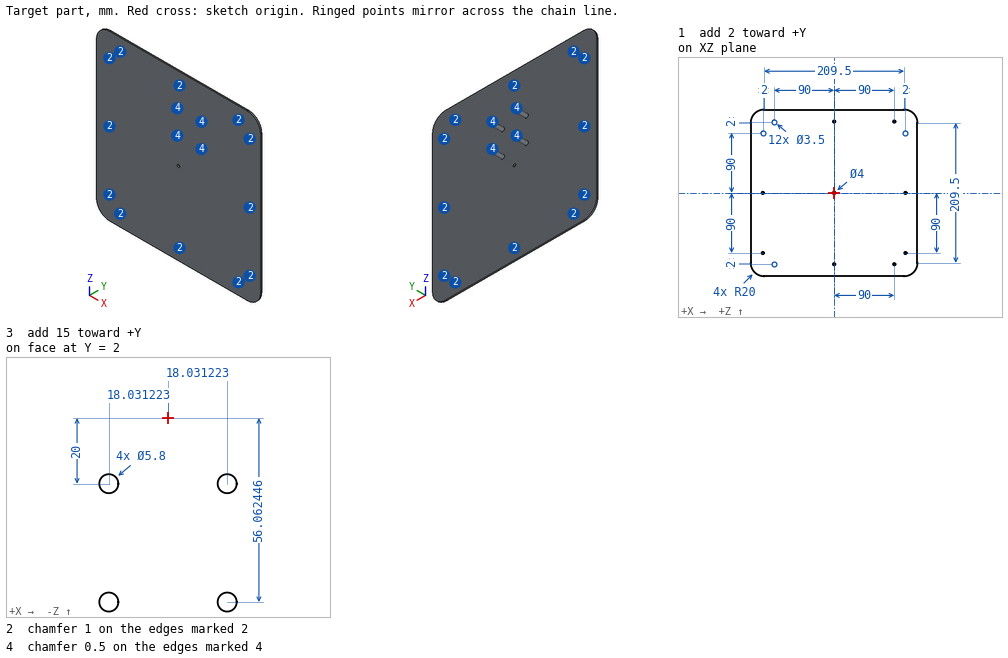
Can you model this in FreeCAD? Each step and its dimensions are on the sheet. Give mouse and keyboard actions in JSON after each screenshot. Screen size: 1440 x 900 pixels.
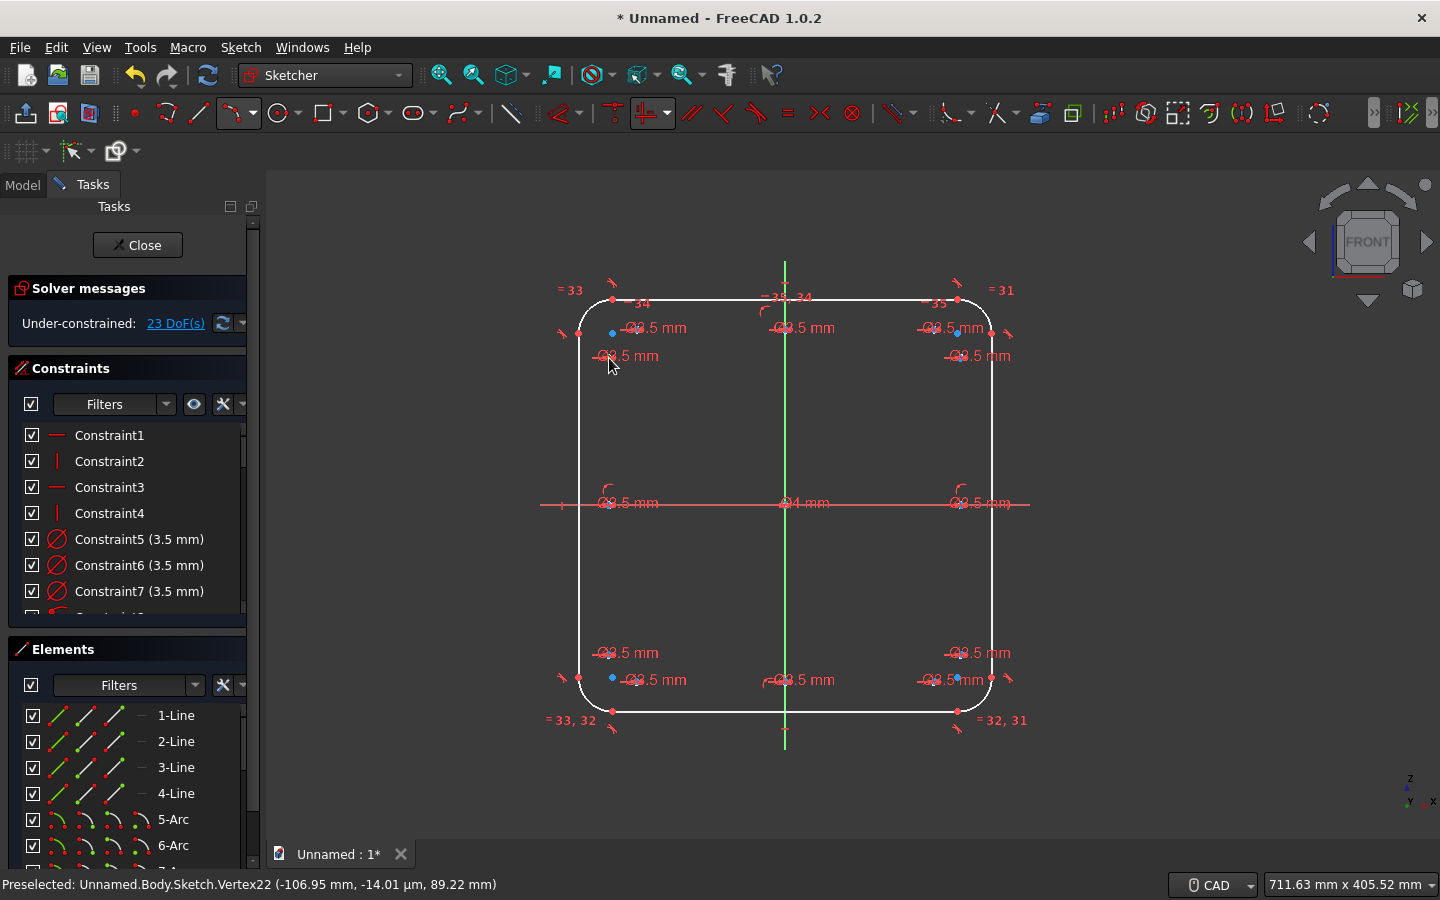
{"action": "left_click", "coordinate": [609, 505]}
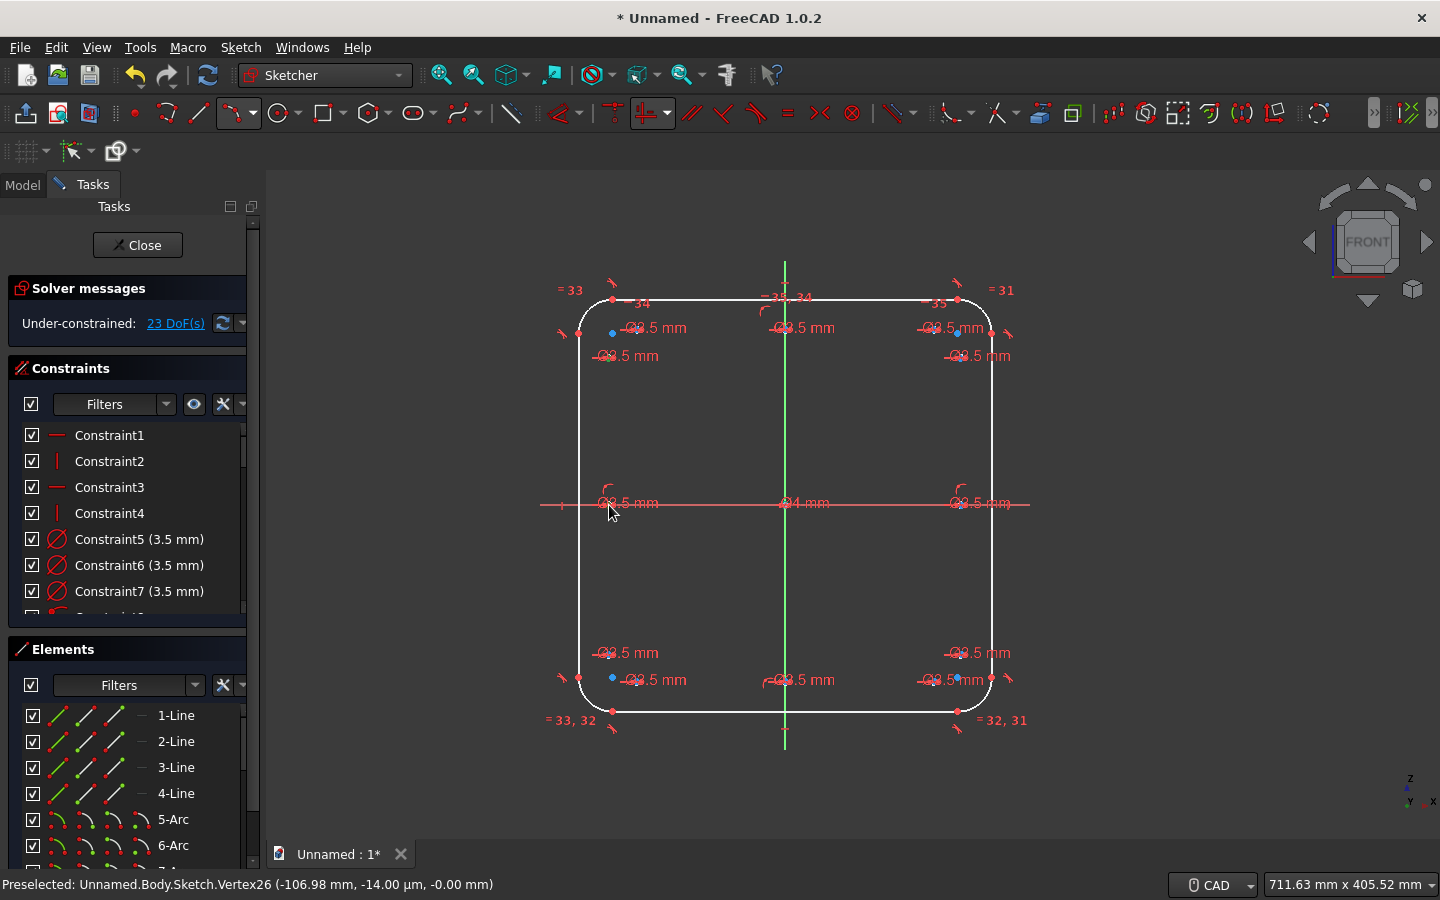
{"action": "left_click", "coordinate": [670, 114]}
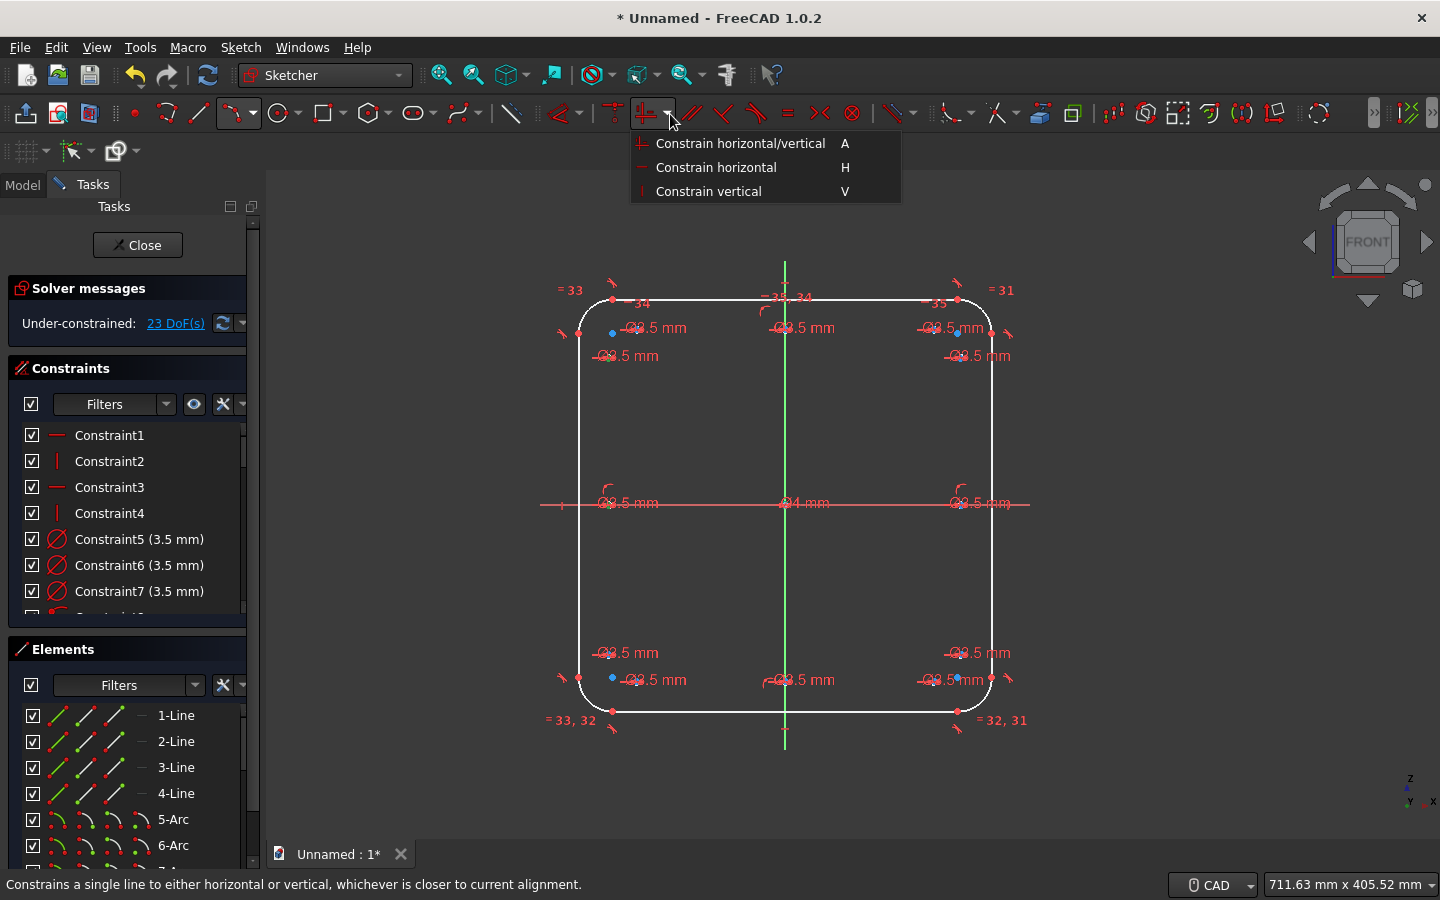
{"action": "left_click", "coordinate": [766, 191]}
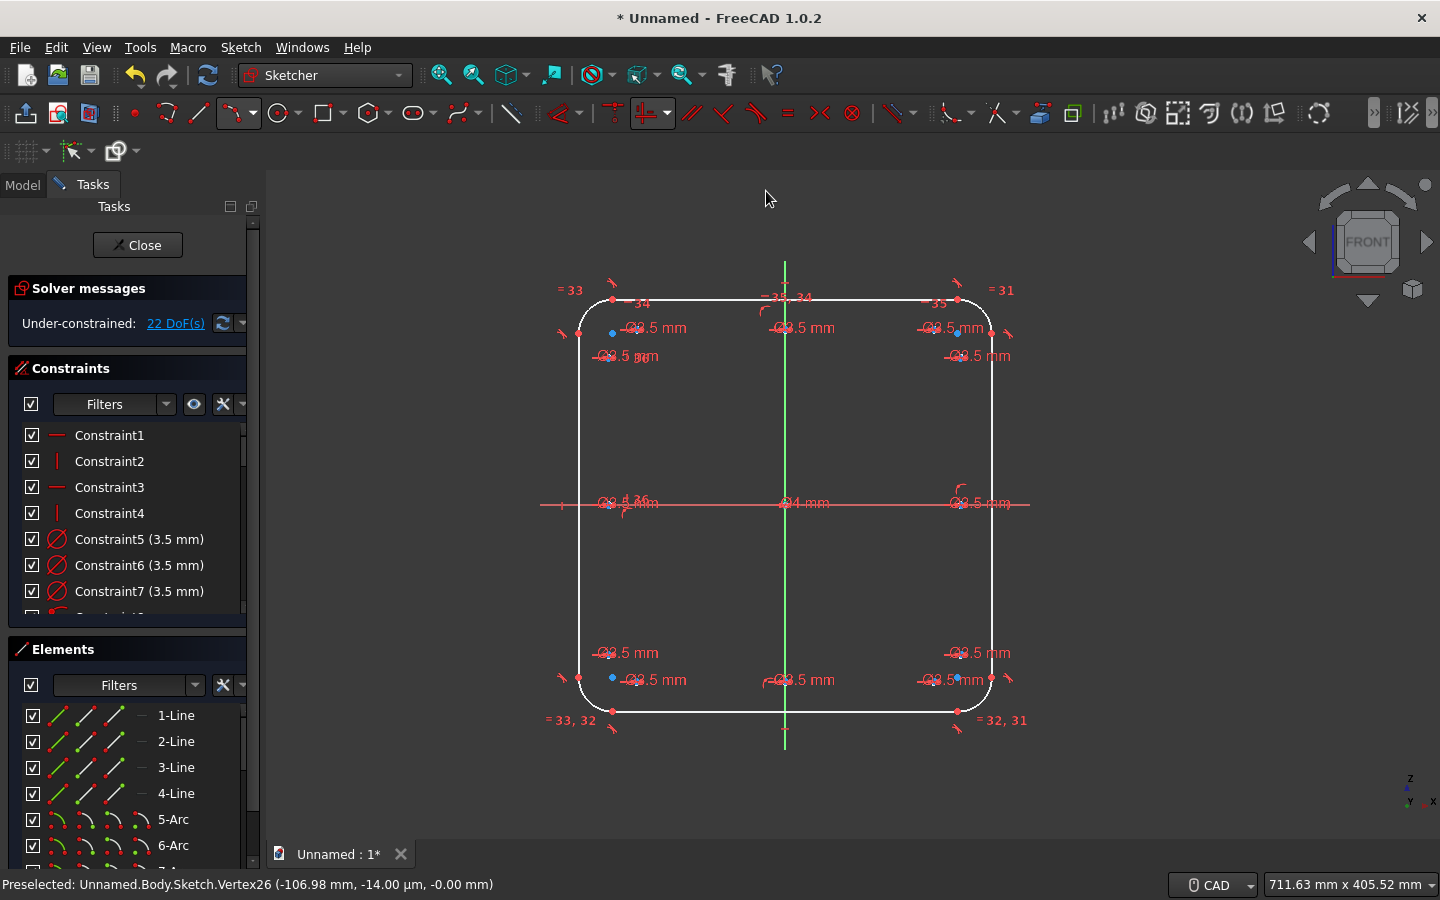
{"action": "left_click", "coordinate": [609, 505]}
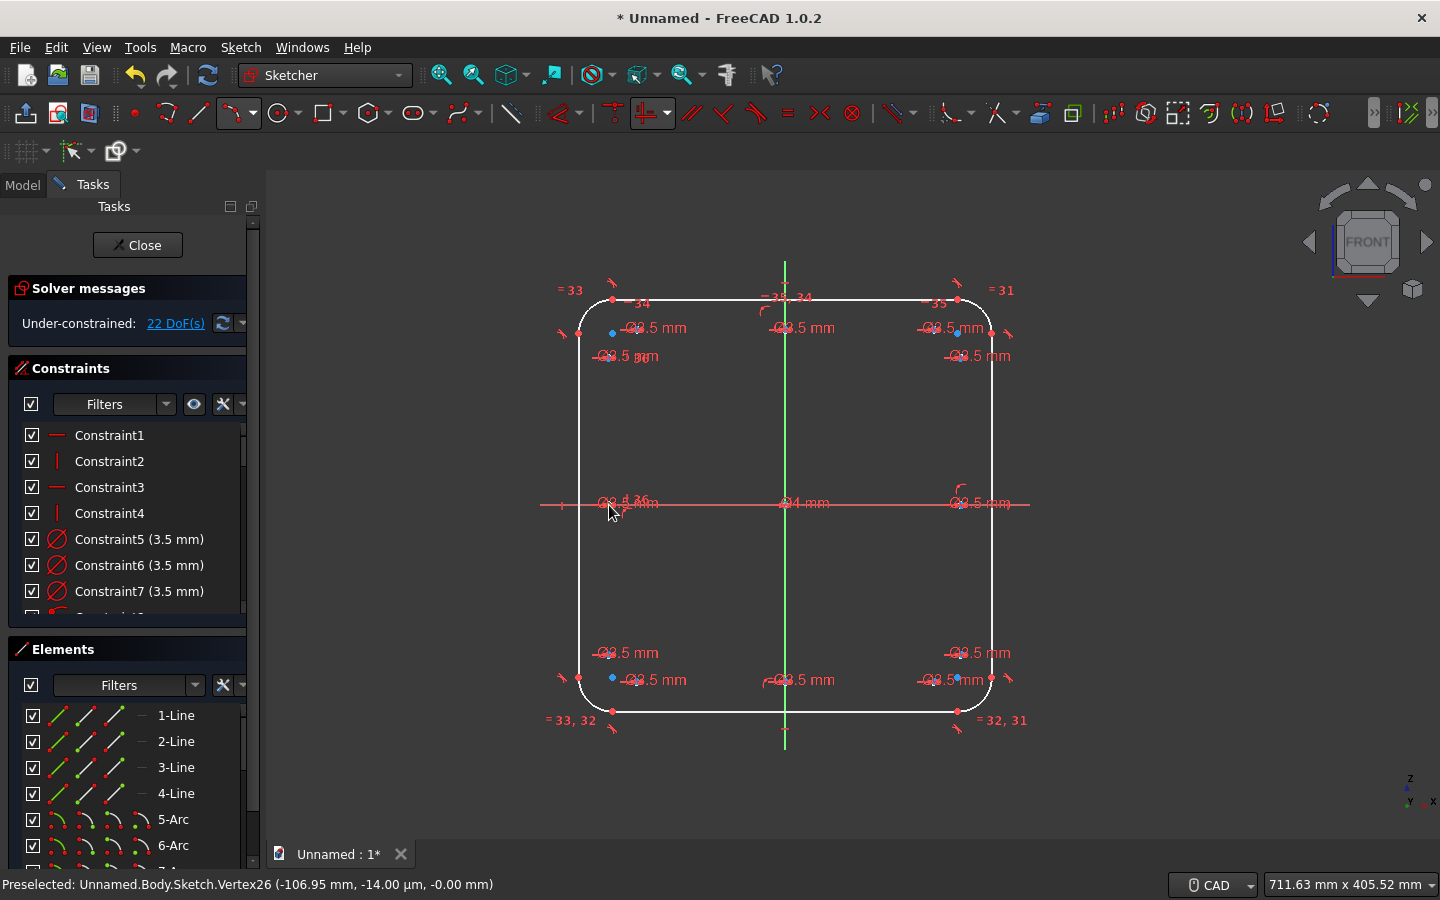
{"action": "left_click", "coordinate": [609, 655]}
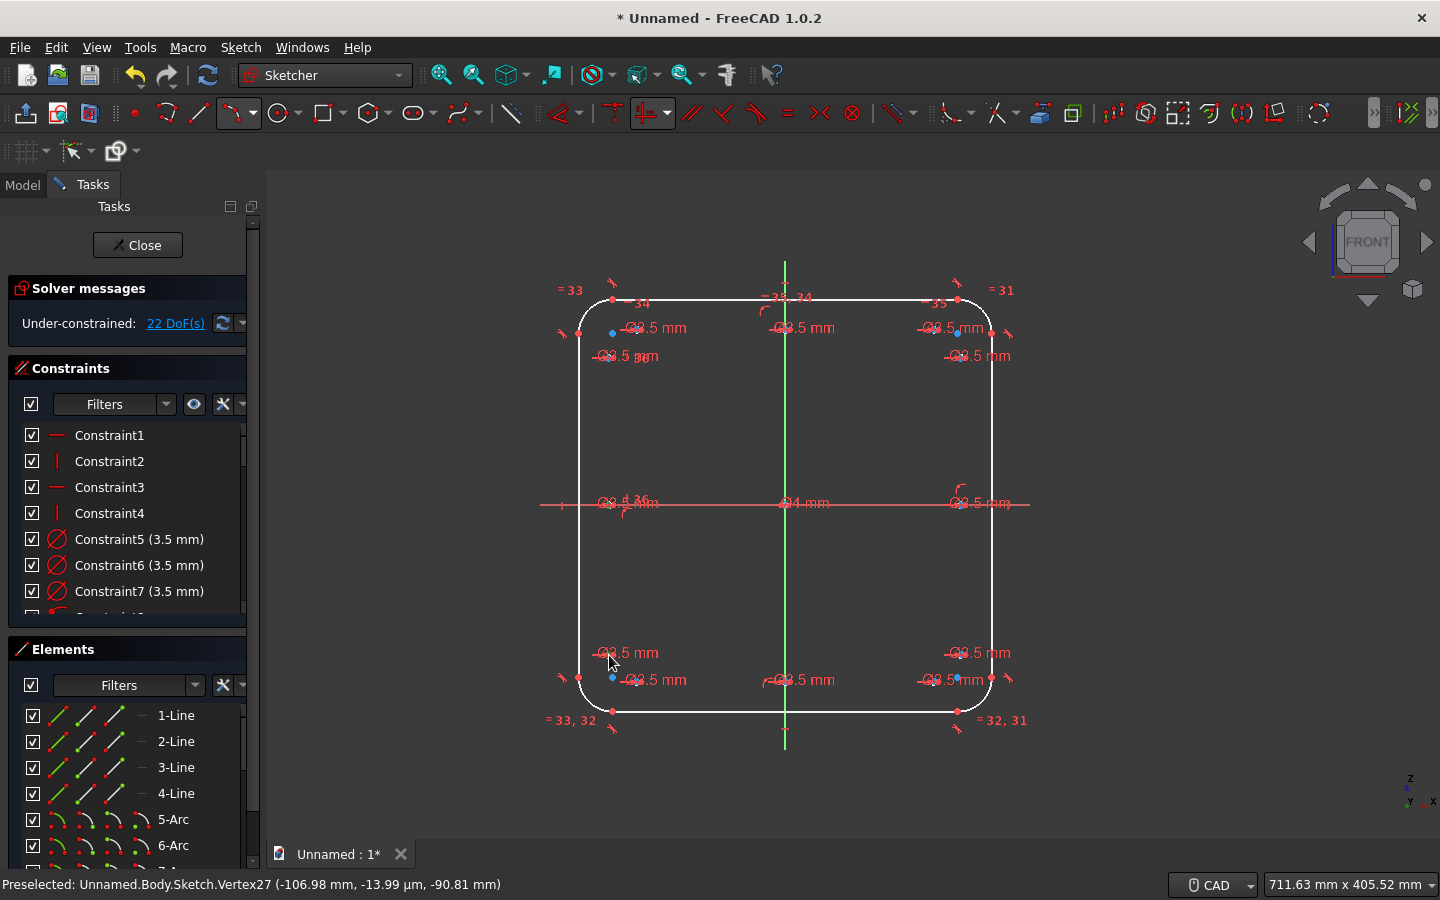
{"action": "left_click", "coordinate": [670, 114]}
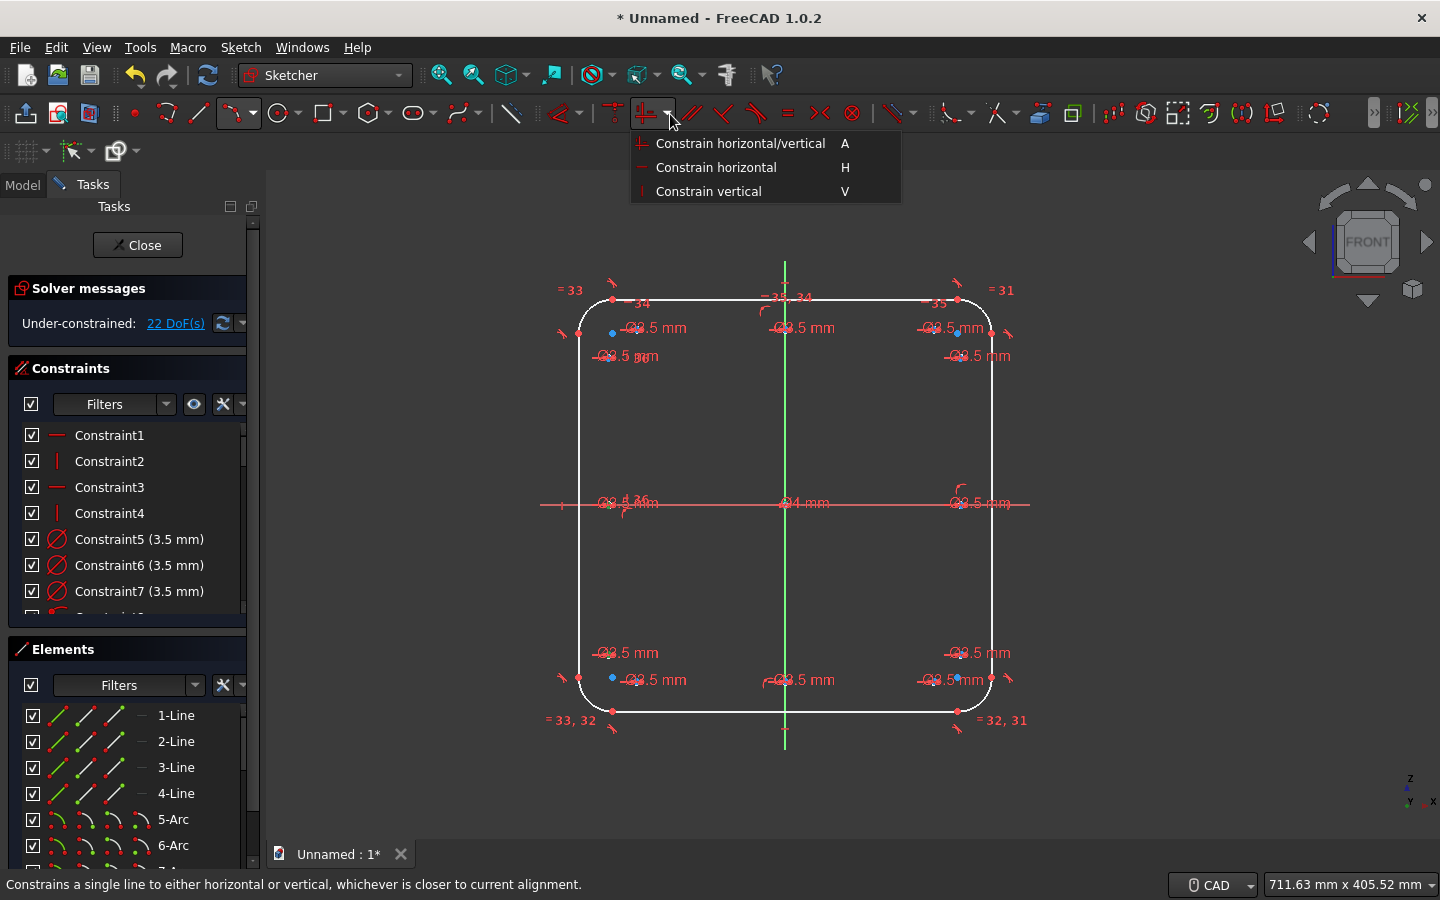
{"action": "left_click", "coordinate": [766, 191]}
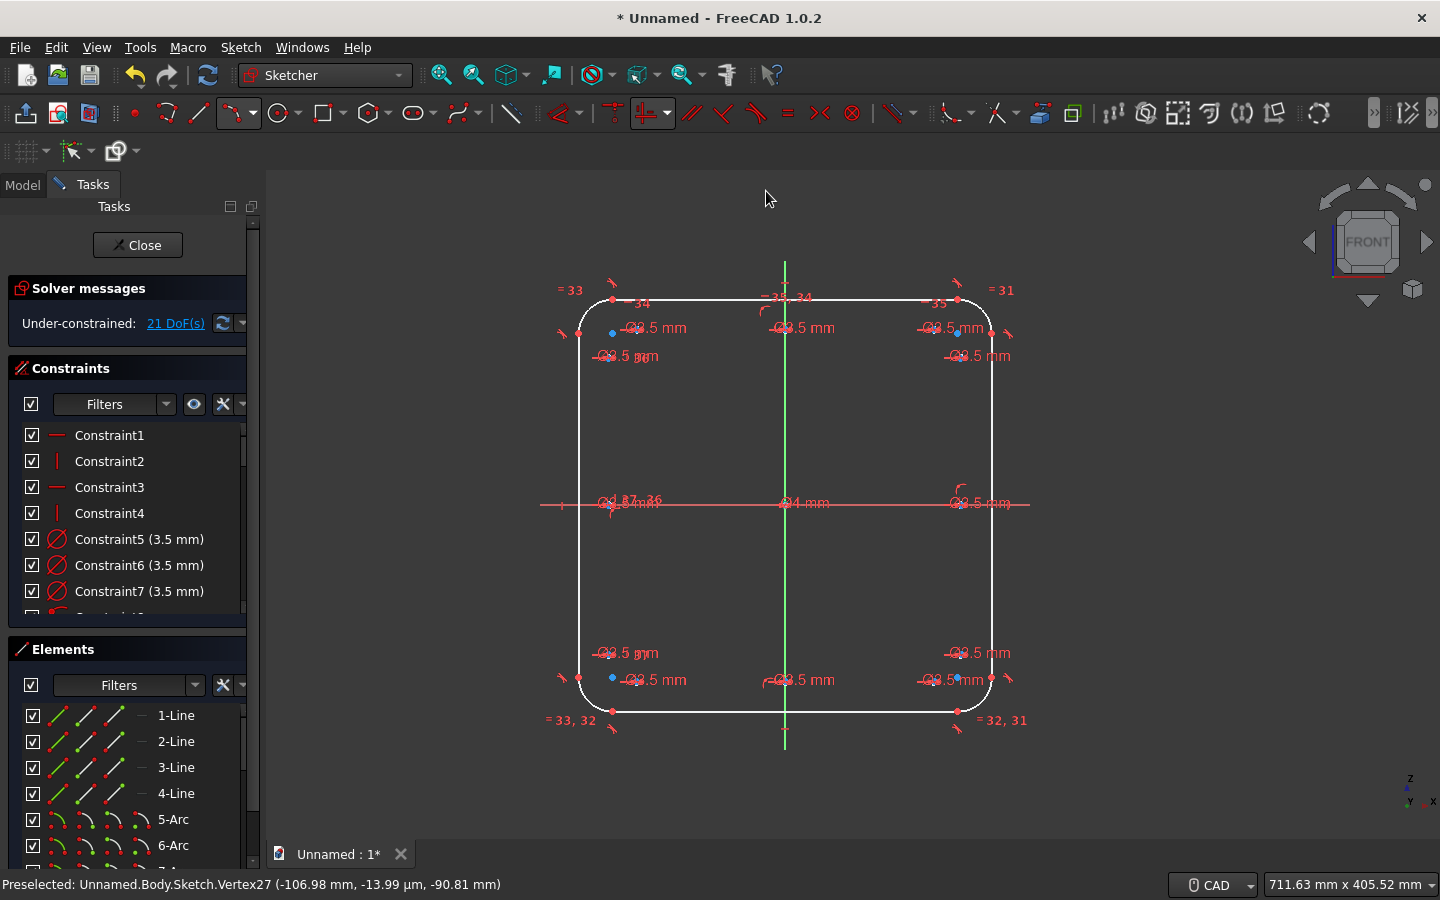
{"action": "left_click", "coordinate": [961, 358]}